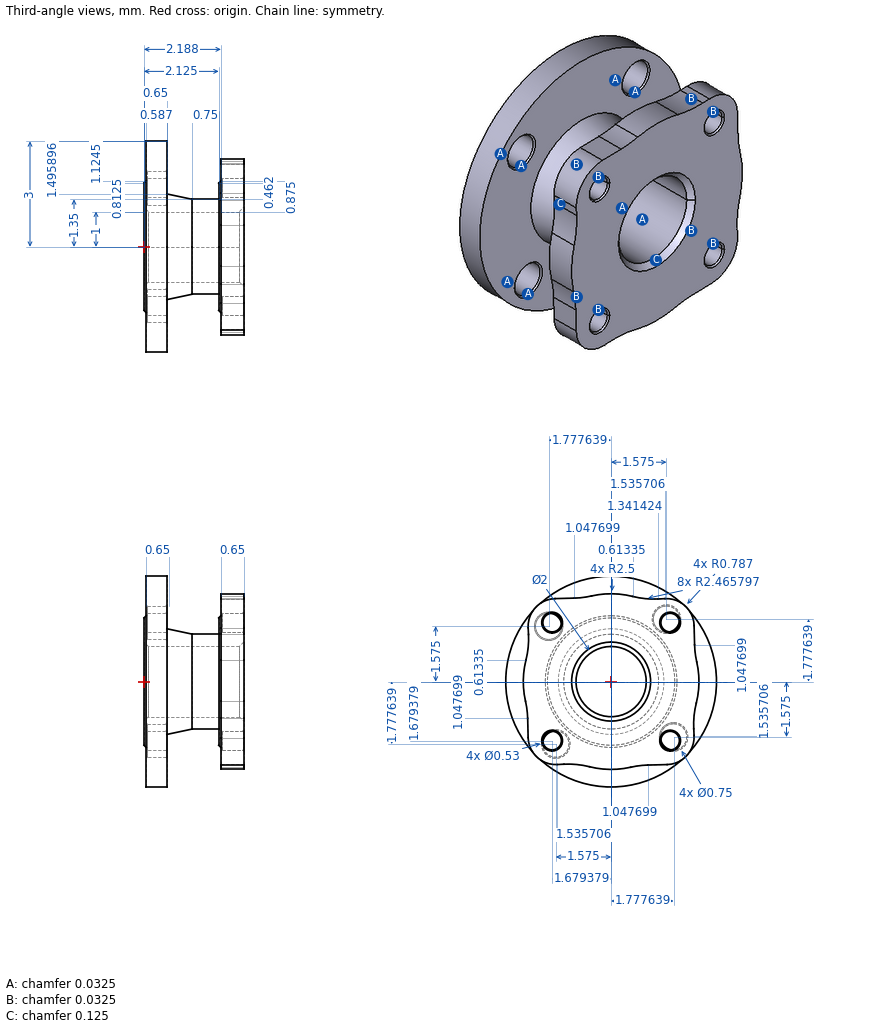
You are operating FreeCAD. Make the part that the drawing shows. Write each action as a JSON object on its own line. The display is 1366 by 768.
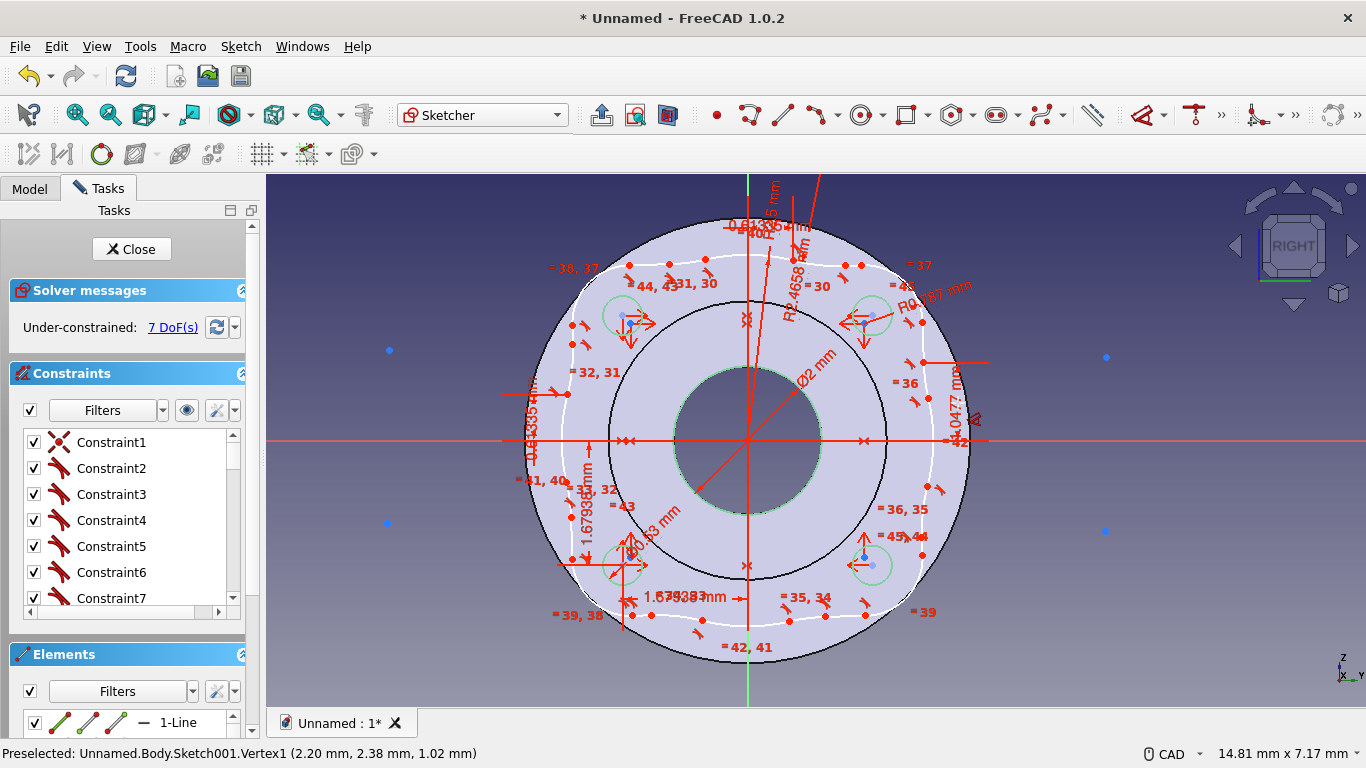
{"action": "left_click", "coordinate": [862, 265]}
{"action": "left_click", "coordinate": [778, 475]}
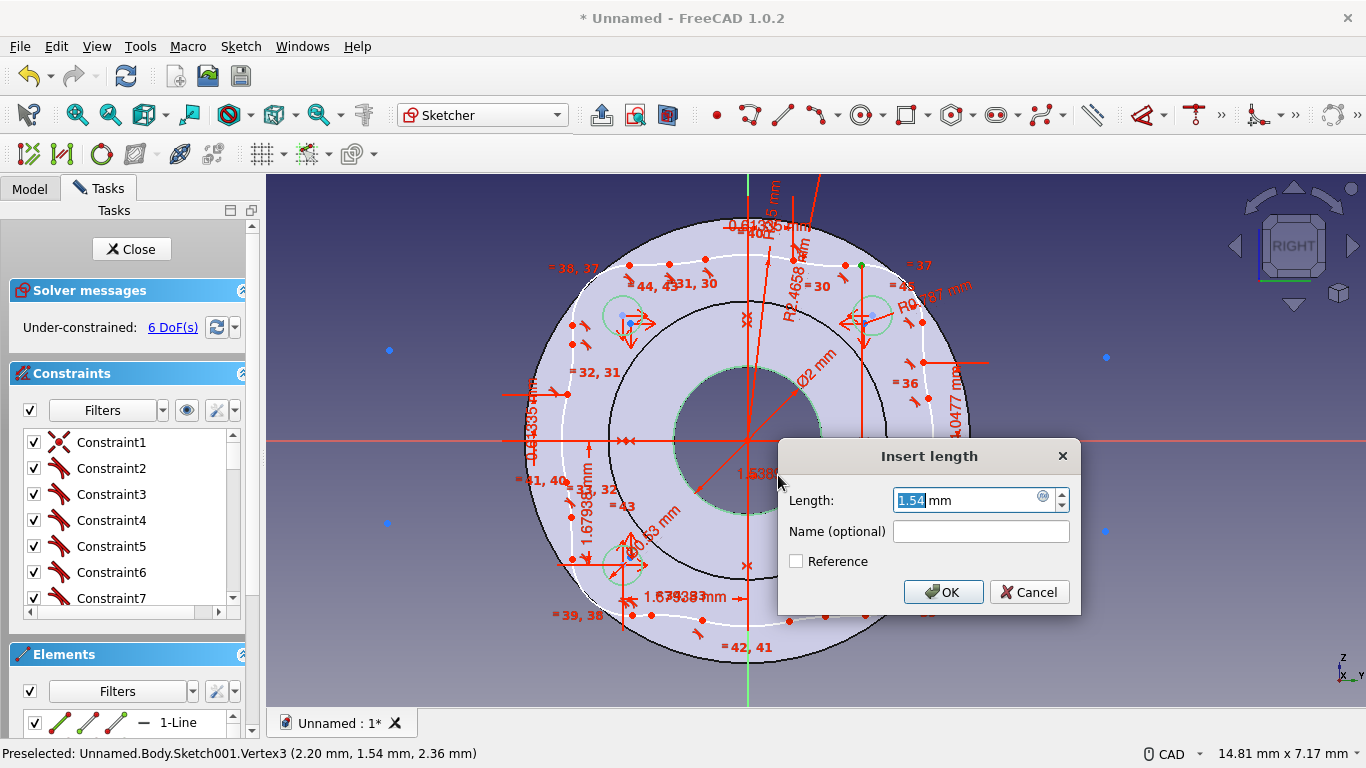
{"action": "type", "text": "1.535706"}
{"action": "key", "text": "Return"}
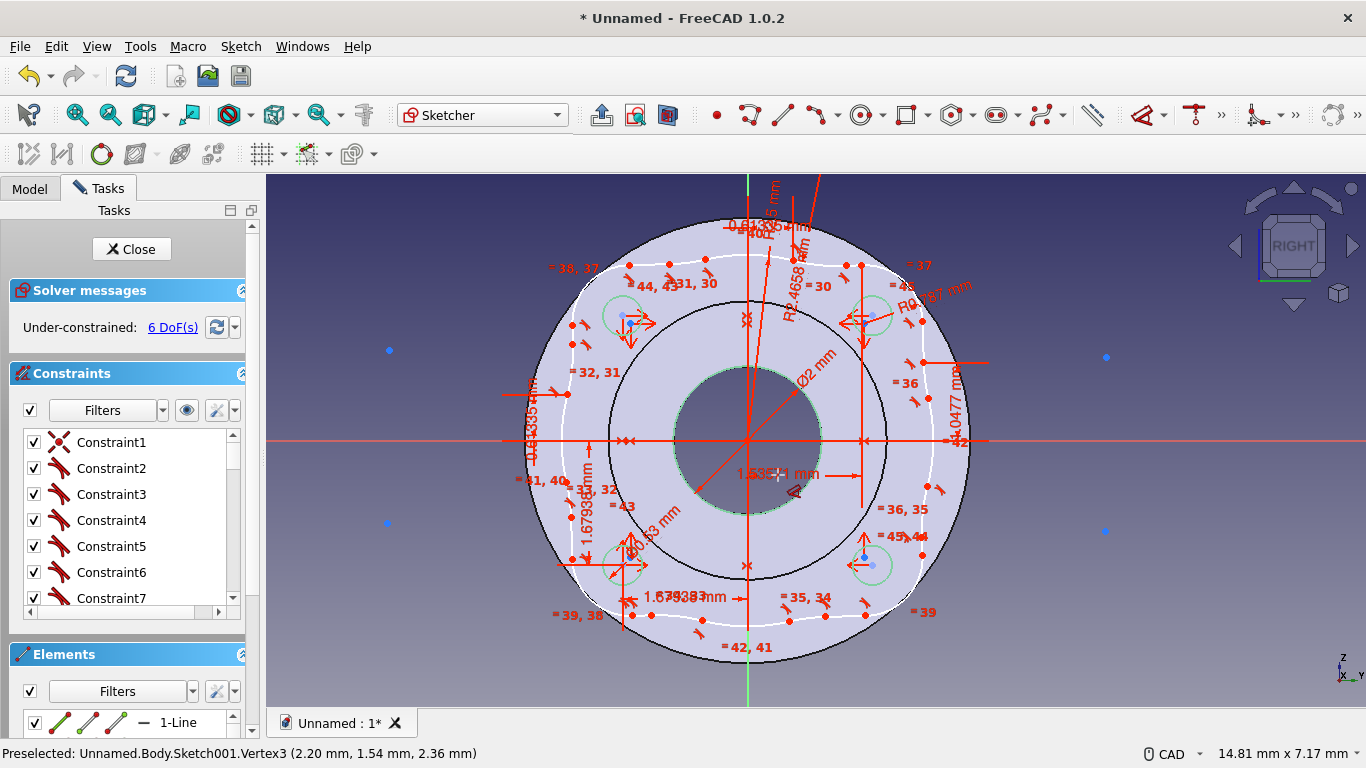
{"action": "left_click", "coordinate": [846, 266]}
{"action": "left_click", "coordinate": [797, 208]}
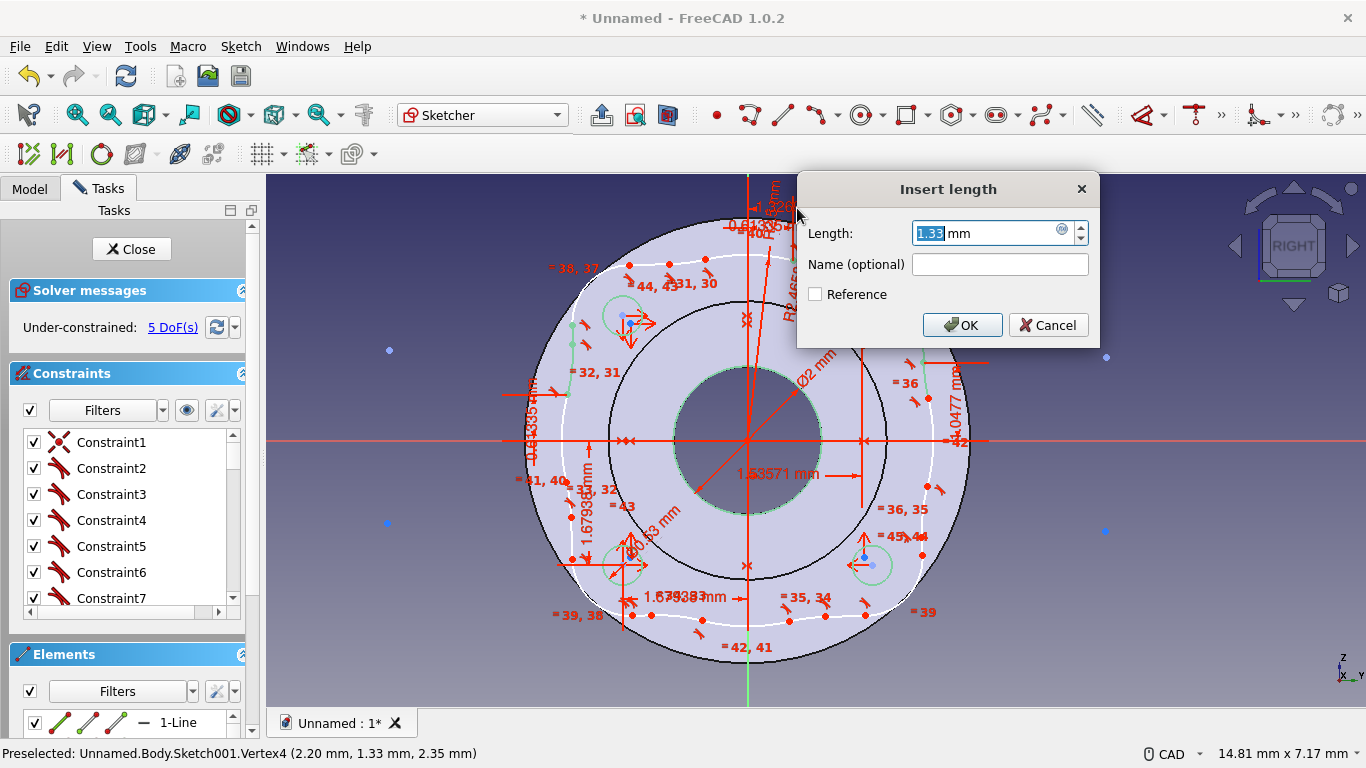
{"action": "type", "text": "1.341424"}
{"action": "key", "text": "Return"}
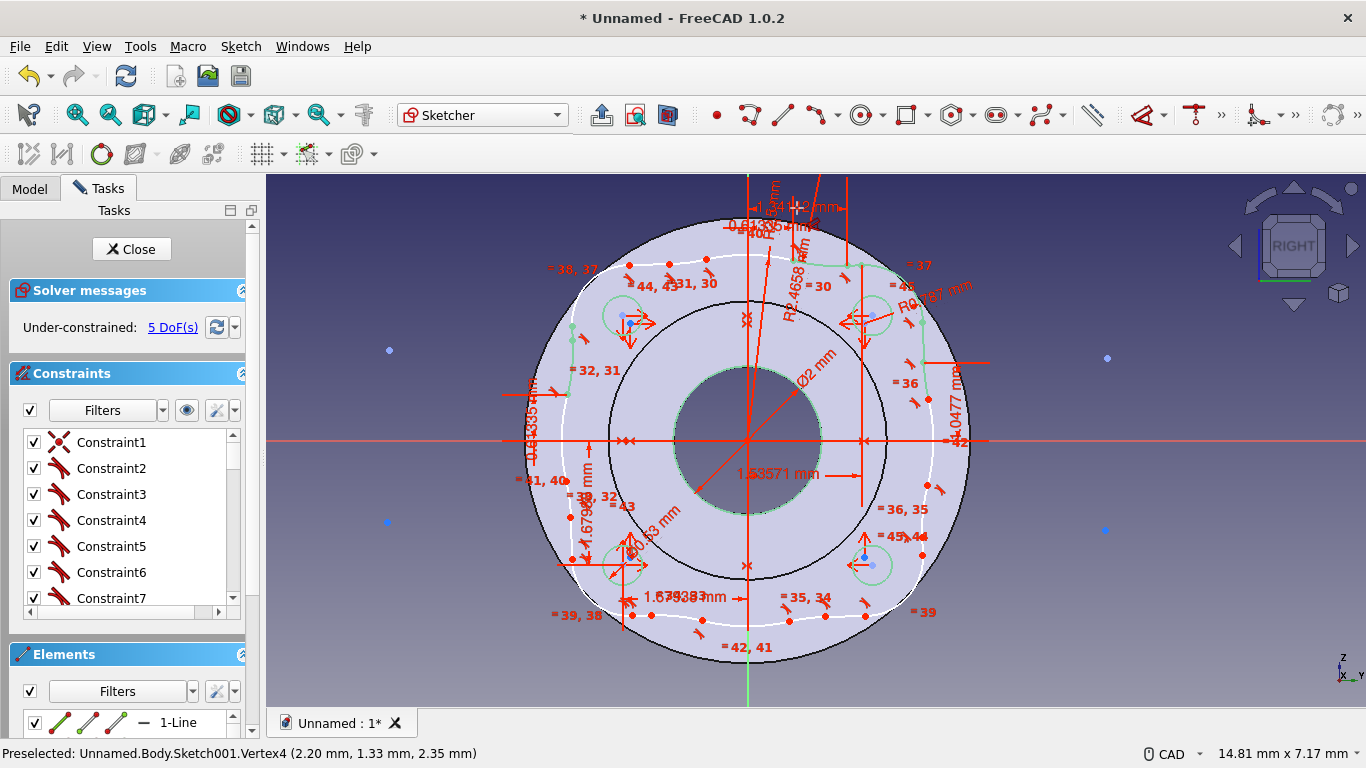
{"action": "left_click", "coordinate": [670, 264]}
{"action": "left_click", "coordinate": [691, 230]}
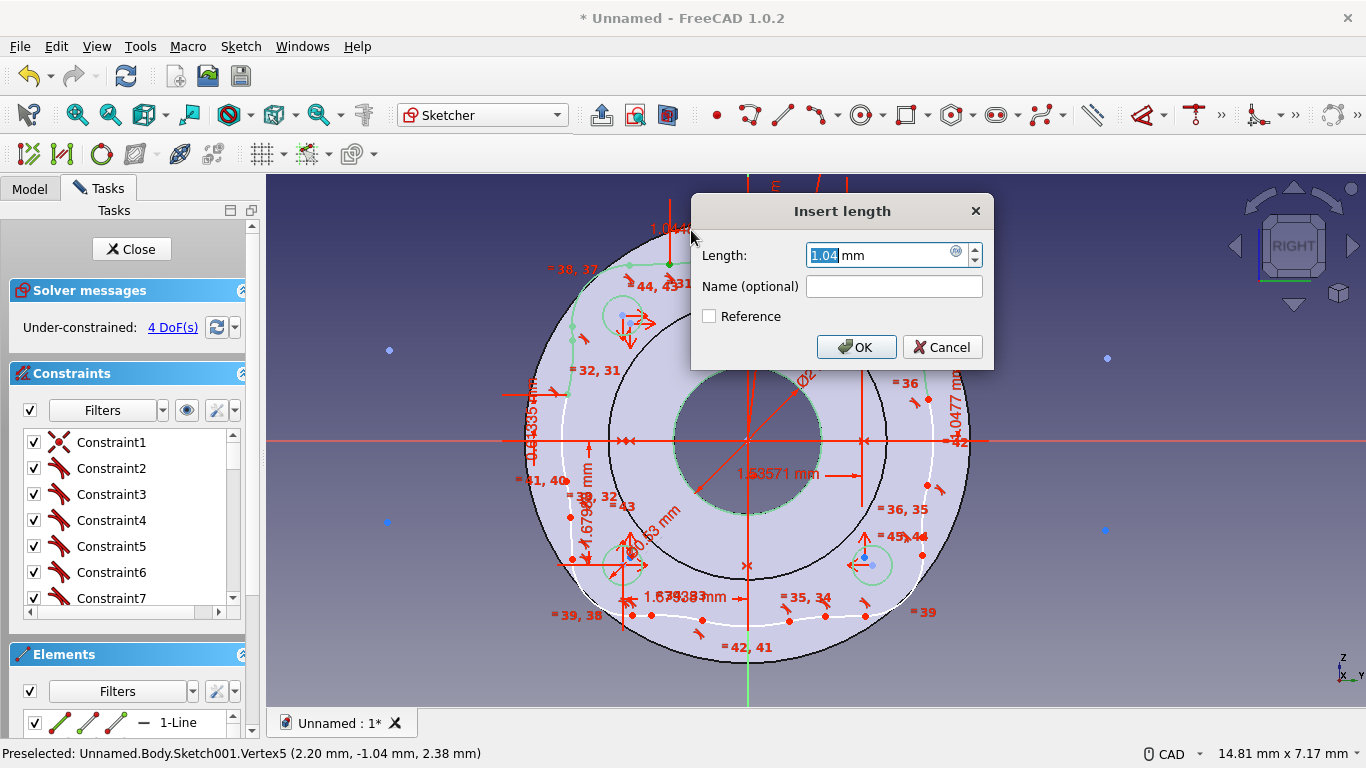
{"action": "type", "text": "1.047699"}
{"action": "key", "text": "Return"}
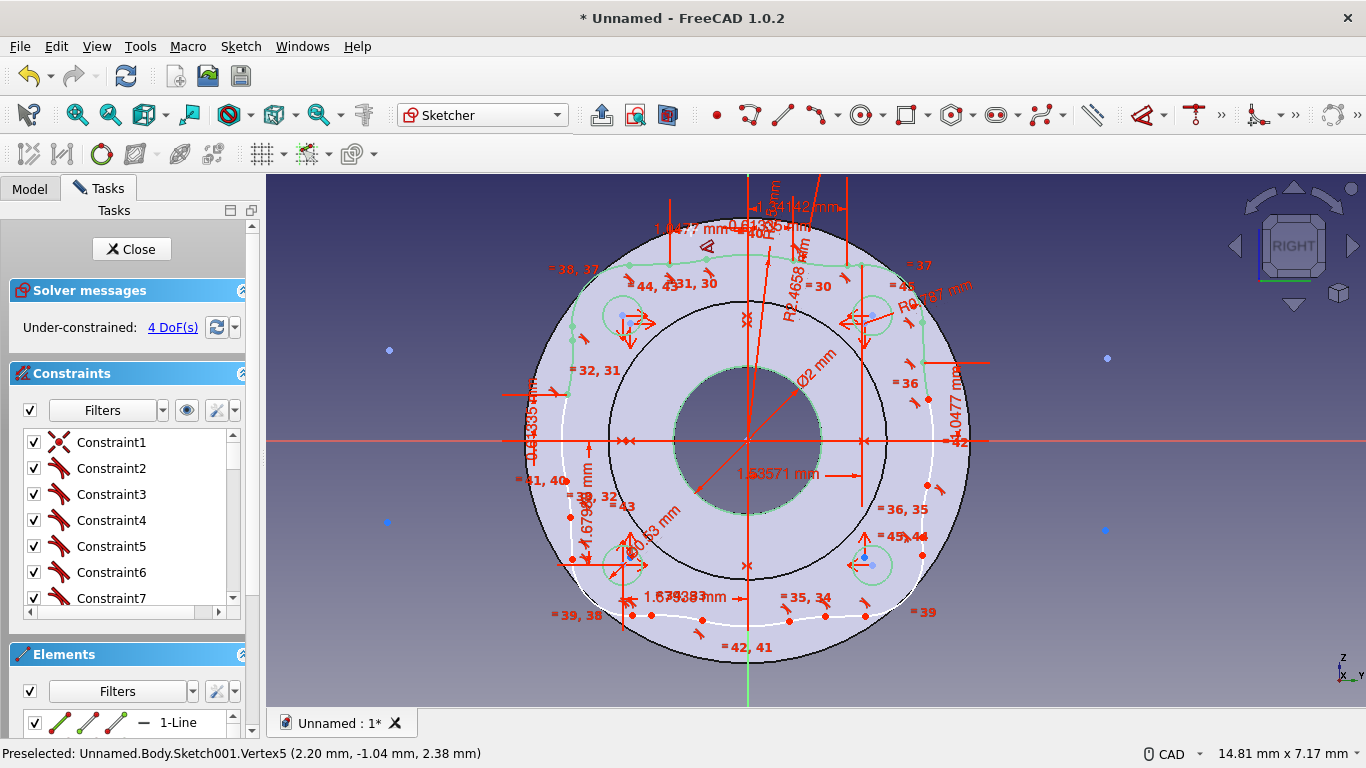
{"action": "left_click", "coordinate": [571, 517]}
{"action": "left_click", "coordinate": [537, 479]}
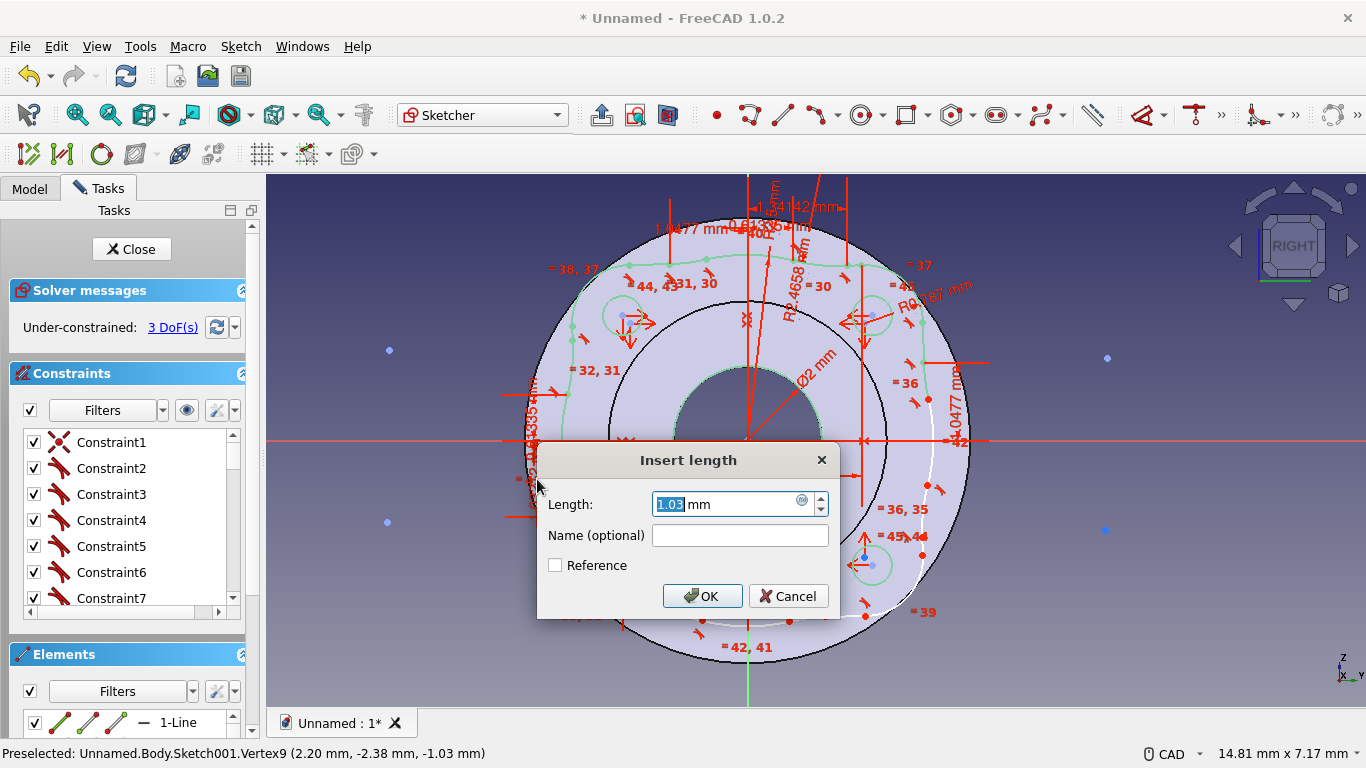
{"action": "type", "text": "1.047699"}
{"action": "key", "text": "Return"}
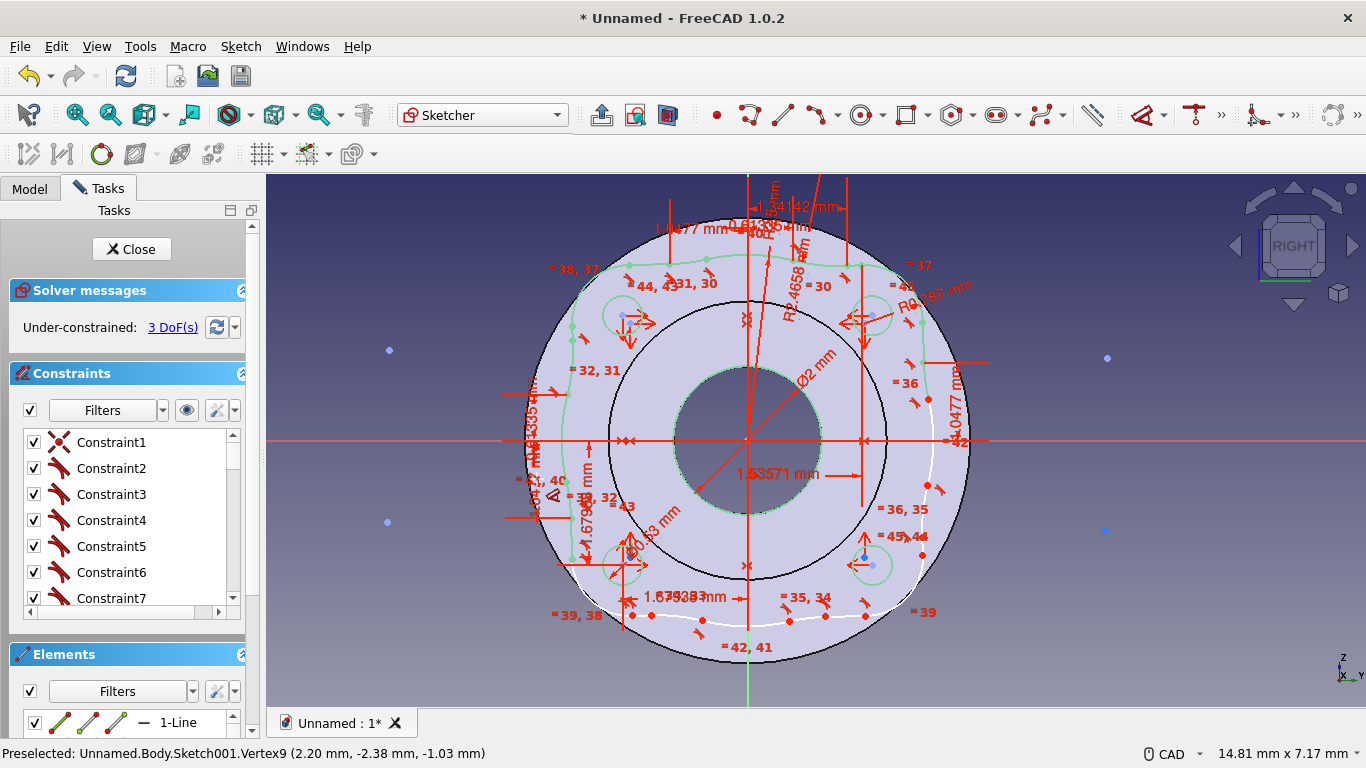
{"action": "left_click", "coordinate": [632, 616]}
{"action": "left_click", "coordinate": [690, 650]}